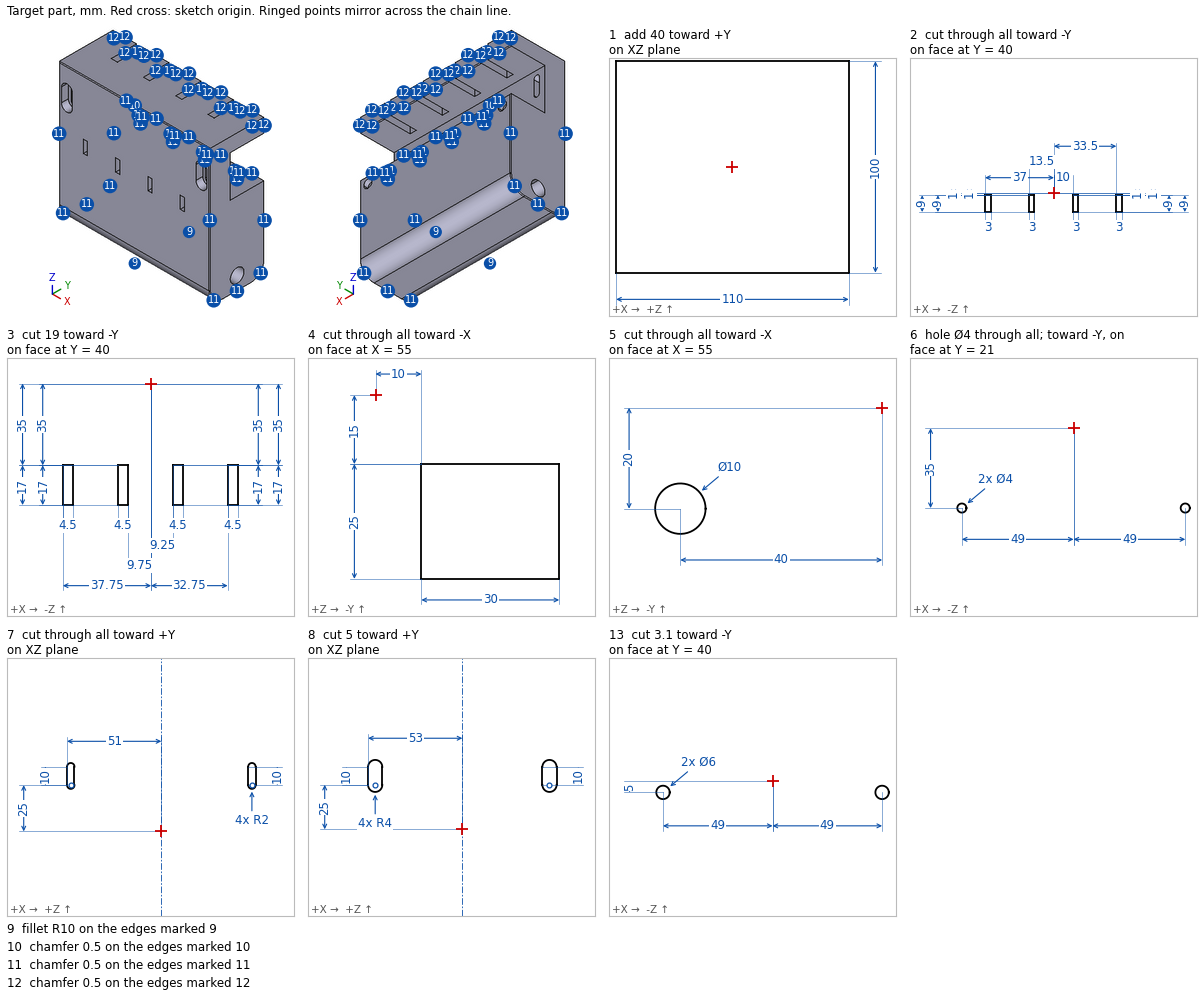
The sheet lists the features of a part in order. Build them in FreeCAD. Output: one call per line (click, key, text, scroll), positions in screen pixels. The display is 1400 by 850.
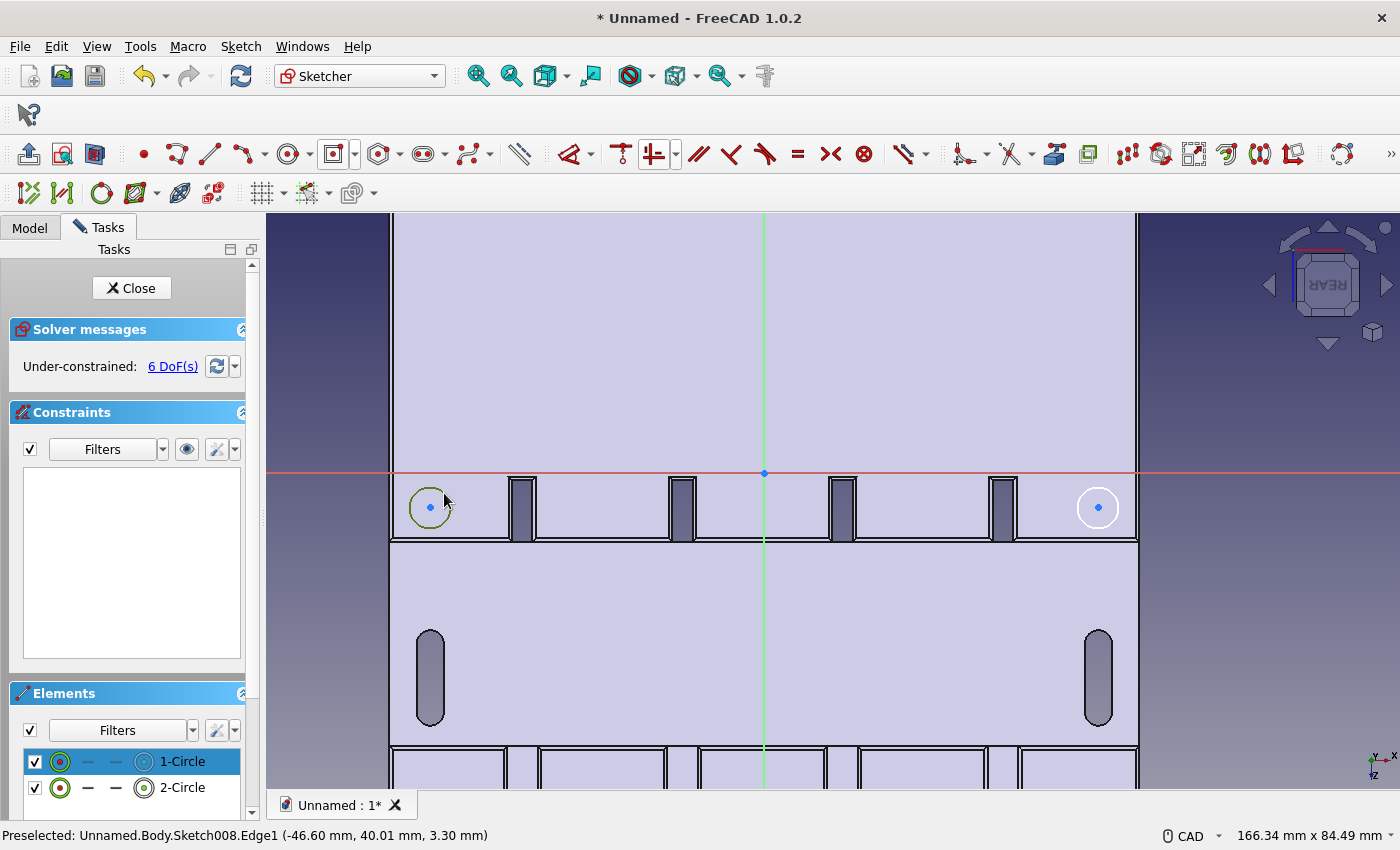
click(1112, 493)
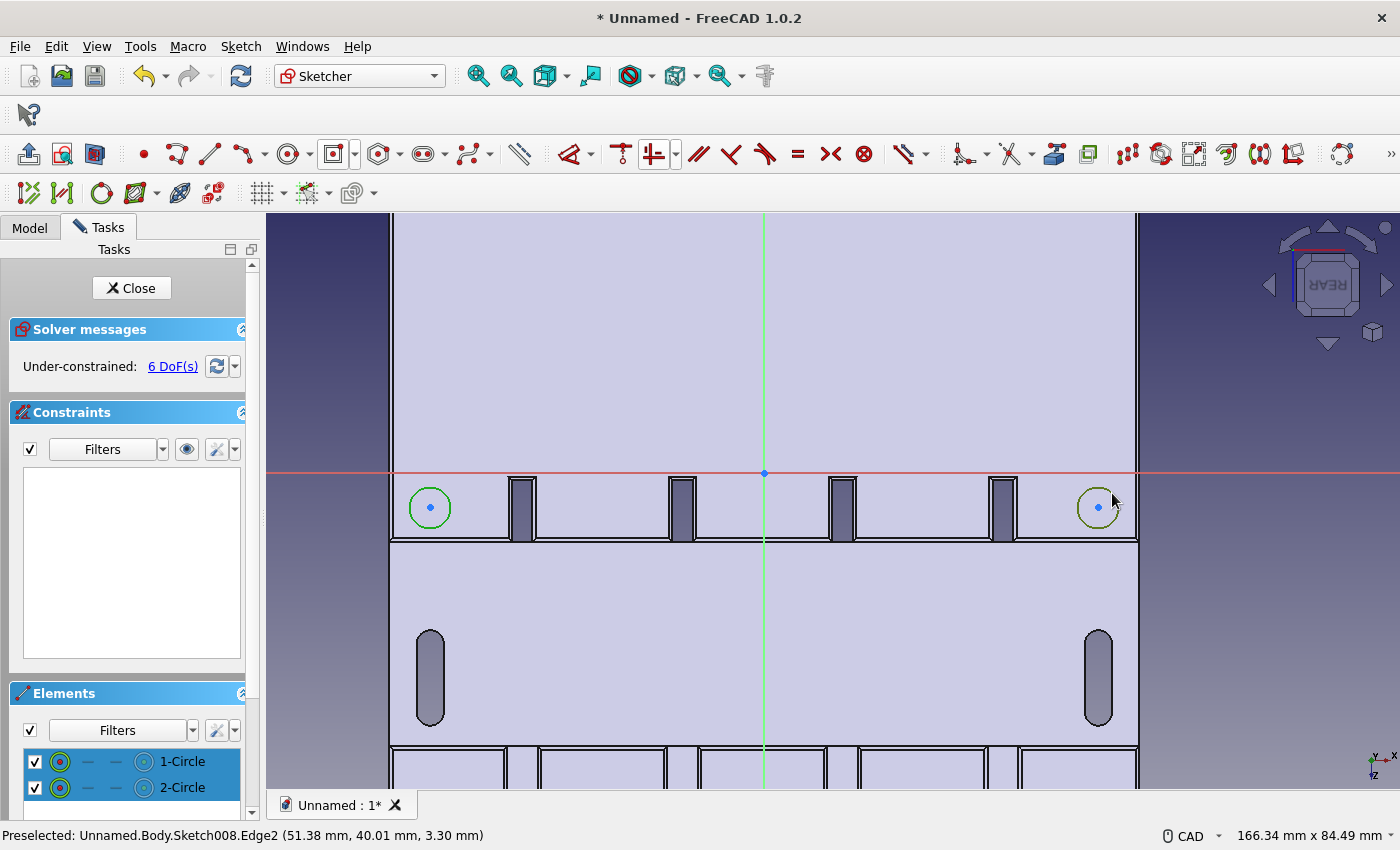
key(e)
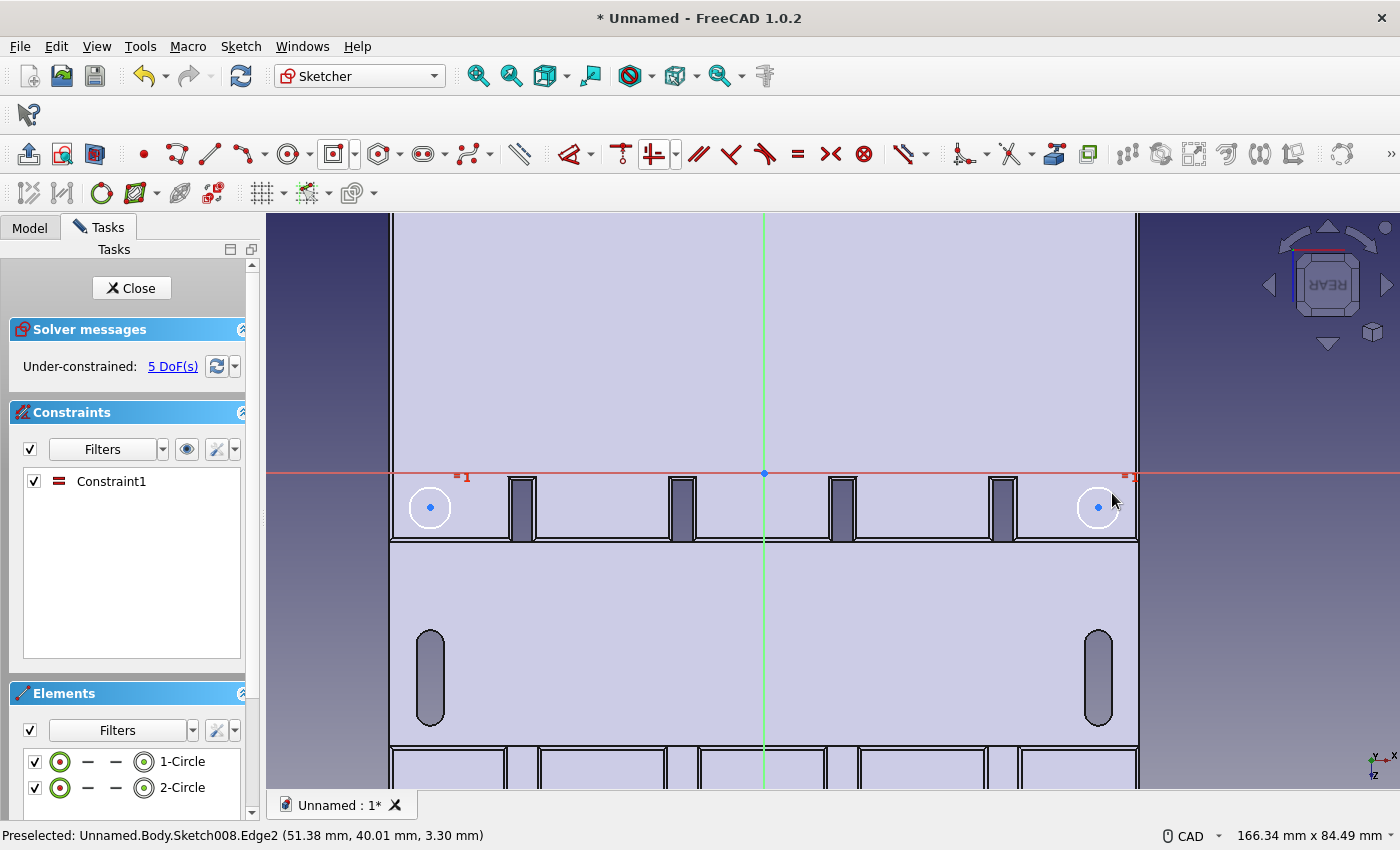
click(430, 508)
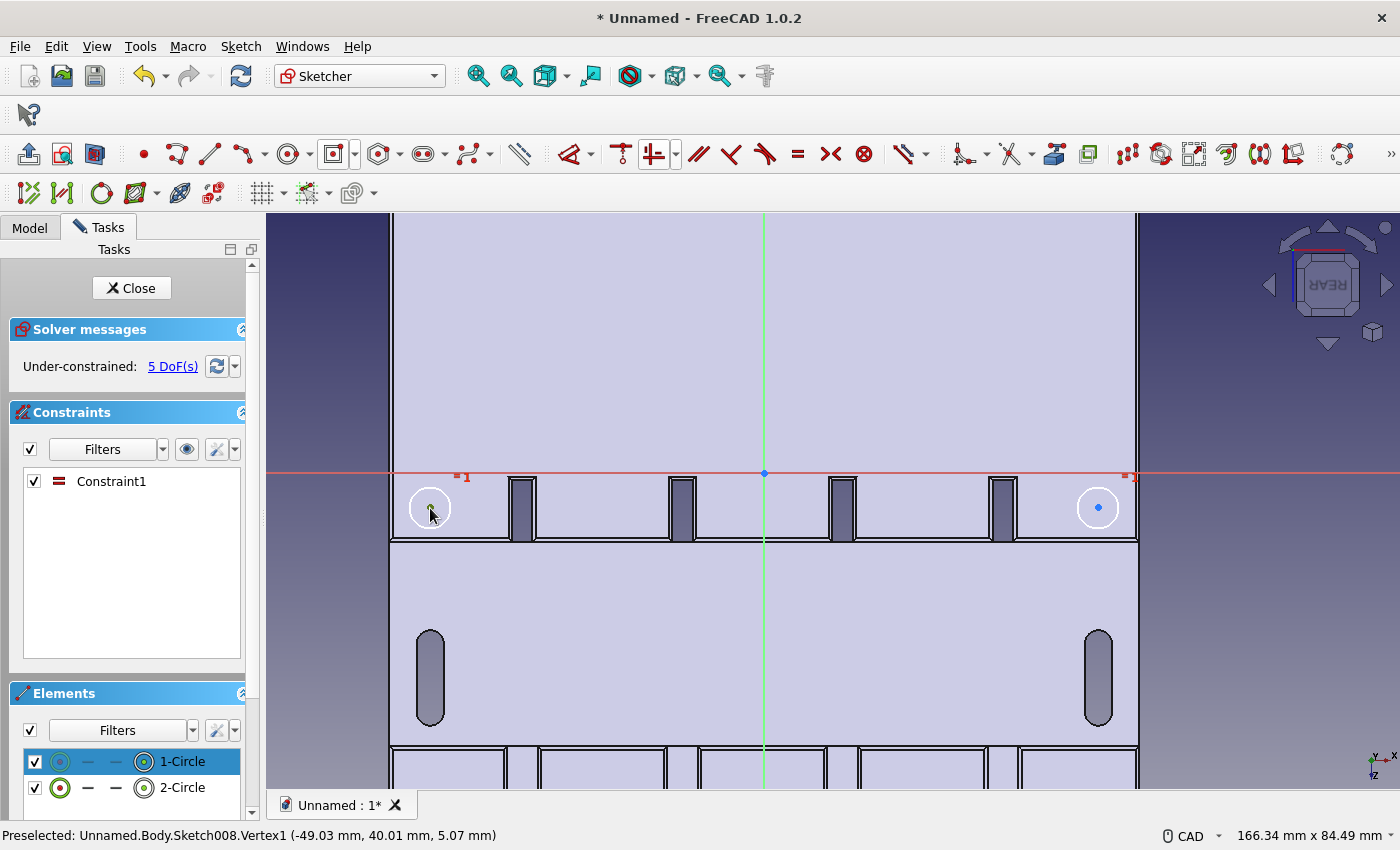
click(1098, 508)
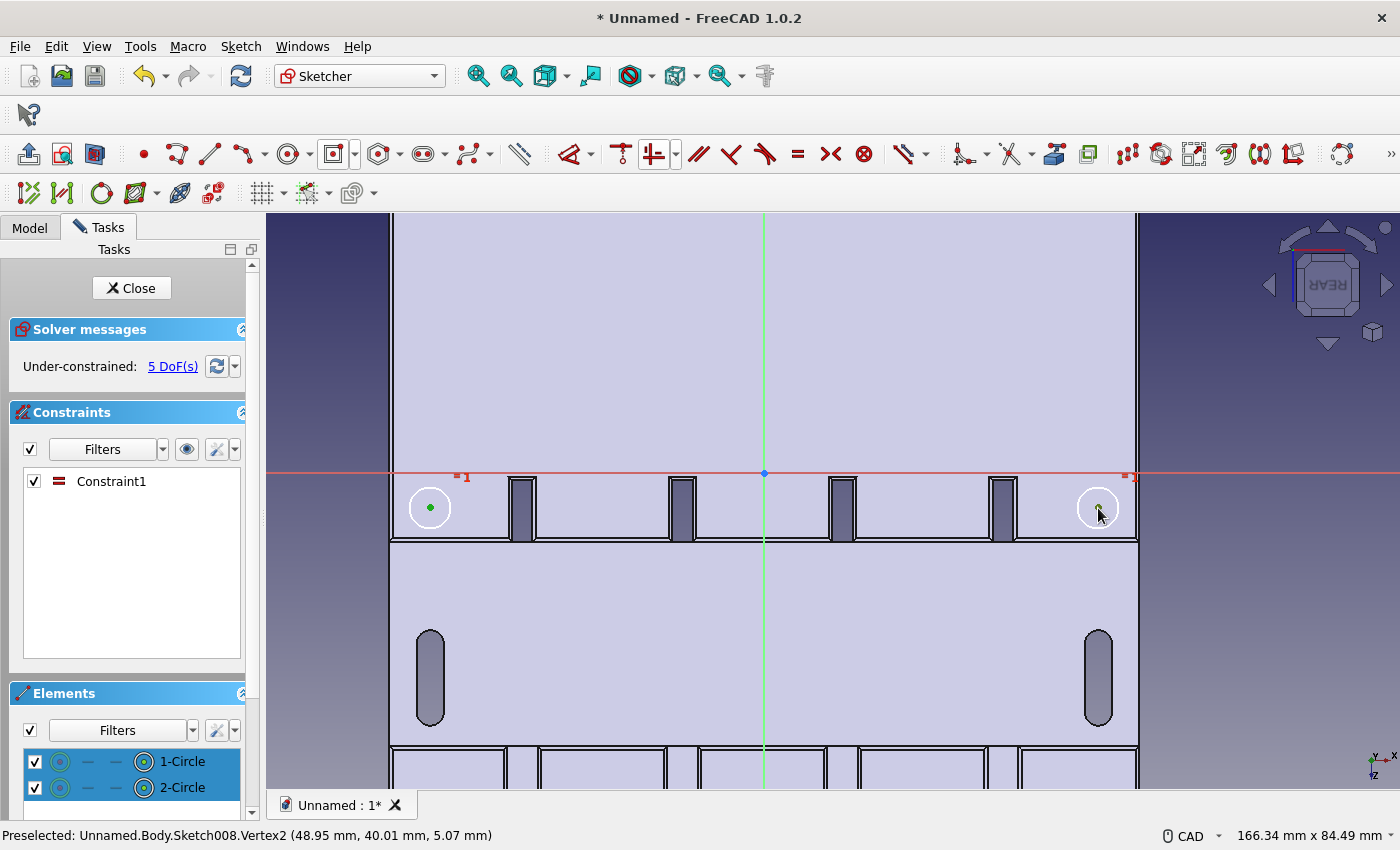
key(h)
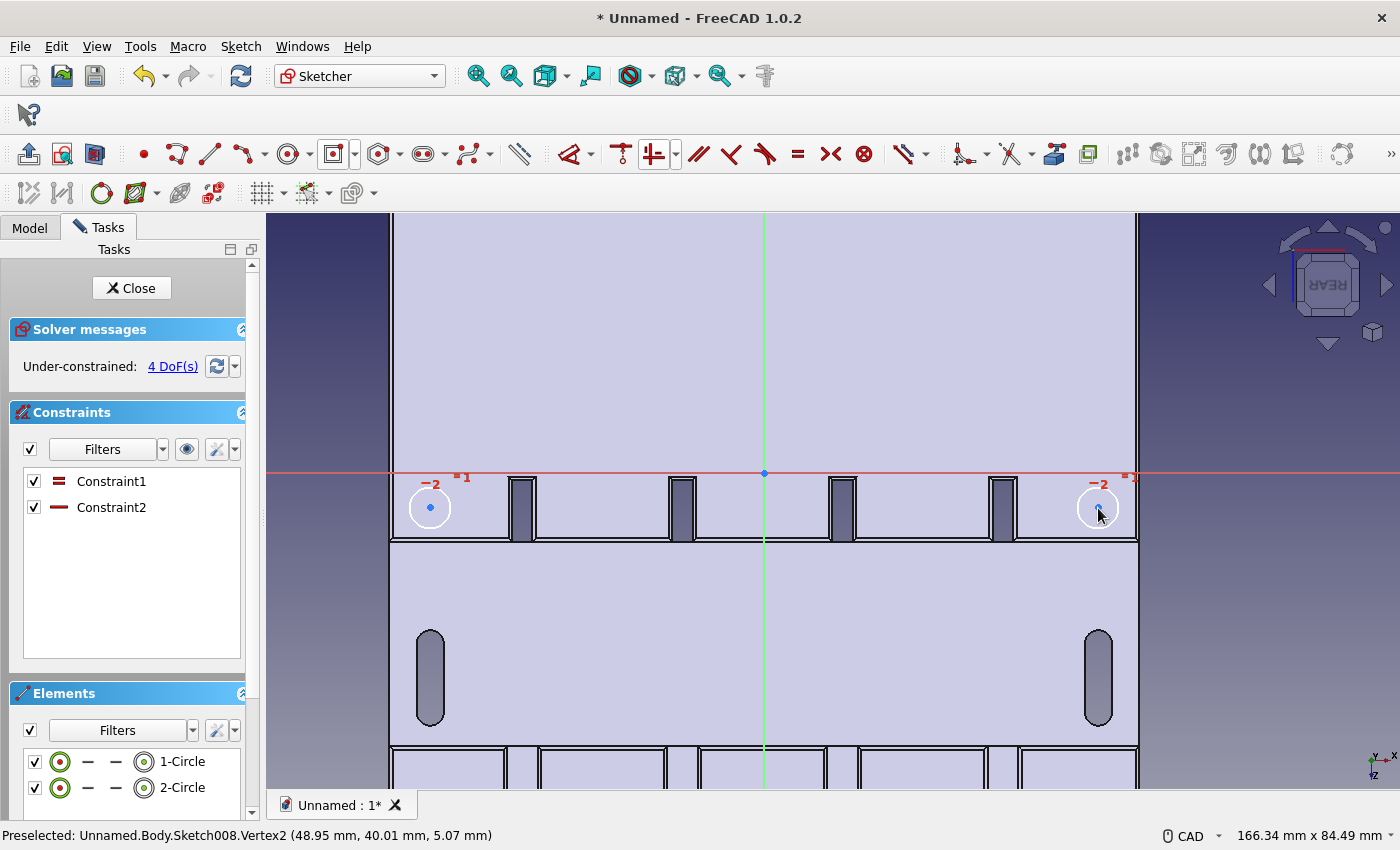
click(568, 154)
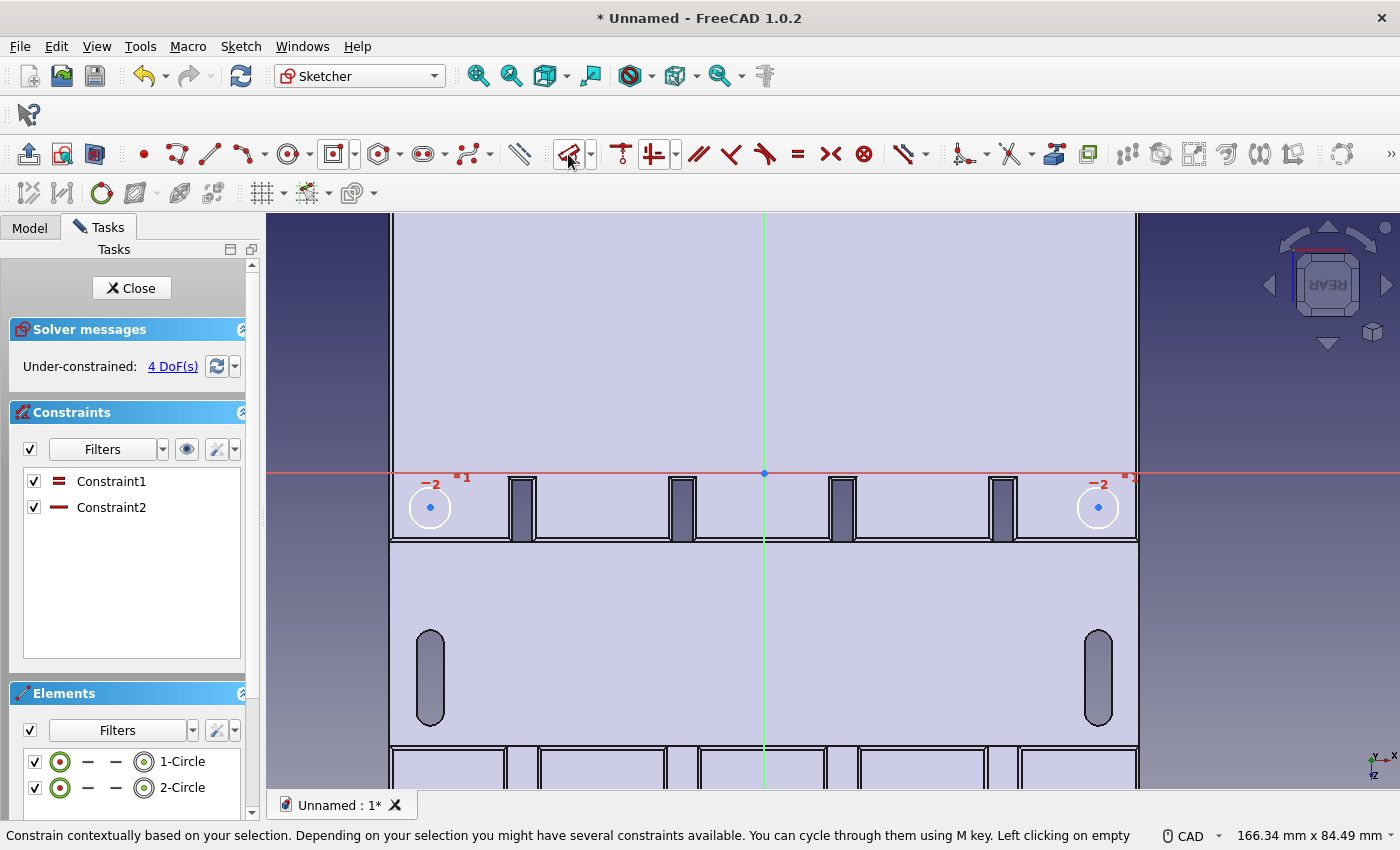
click(444, 493)
click(480, 491)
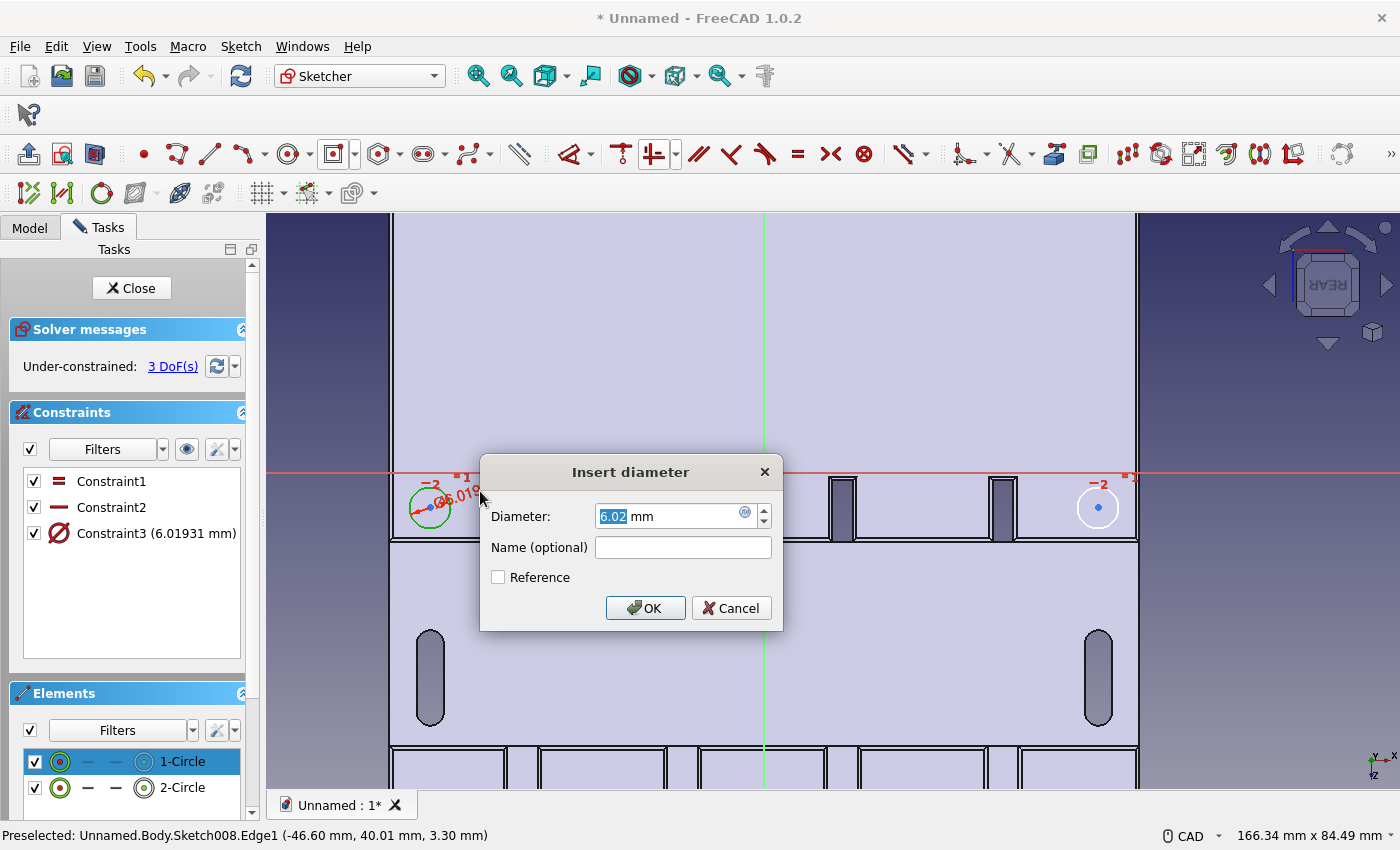
text(6)
key(Return)